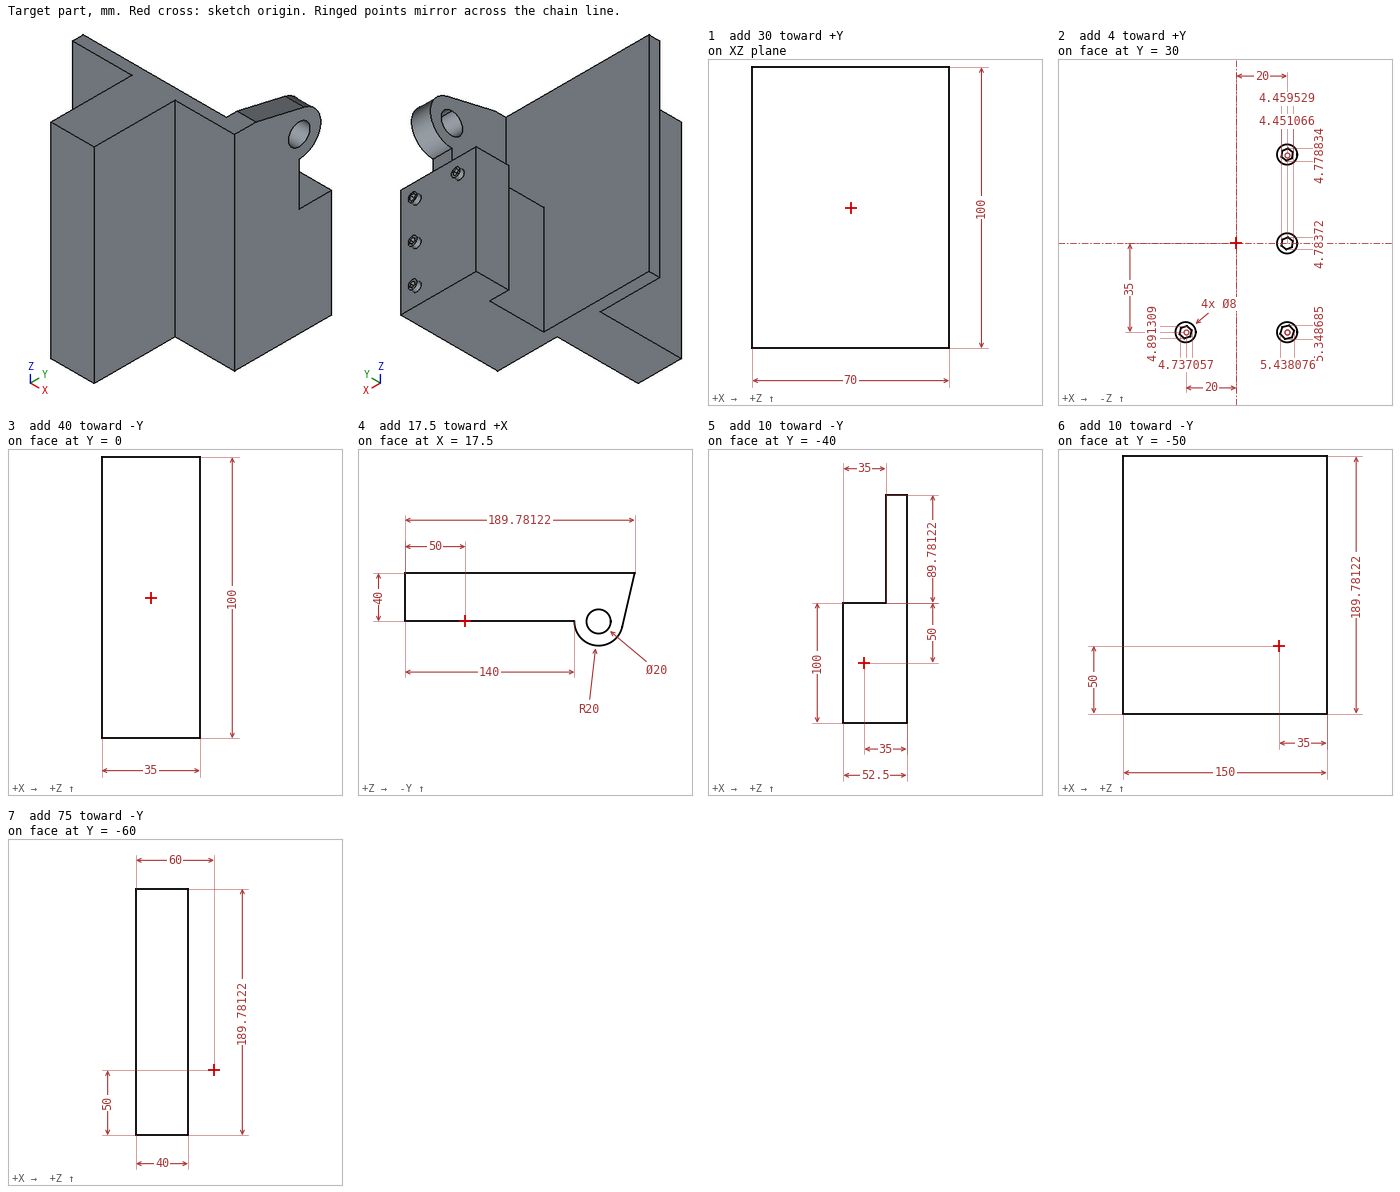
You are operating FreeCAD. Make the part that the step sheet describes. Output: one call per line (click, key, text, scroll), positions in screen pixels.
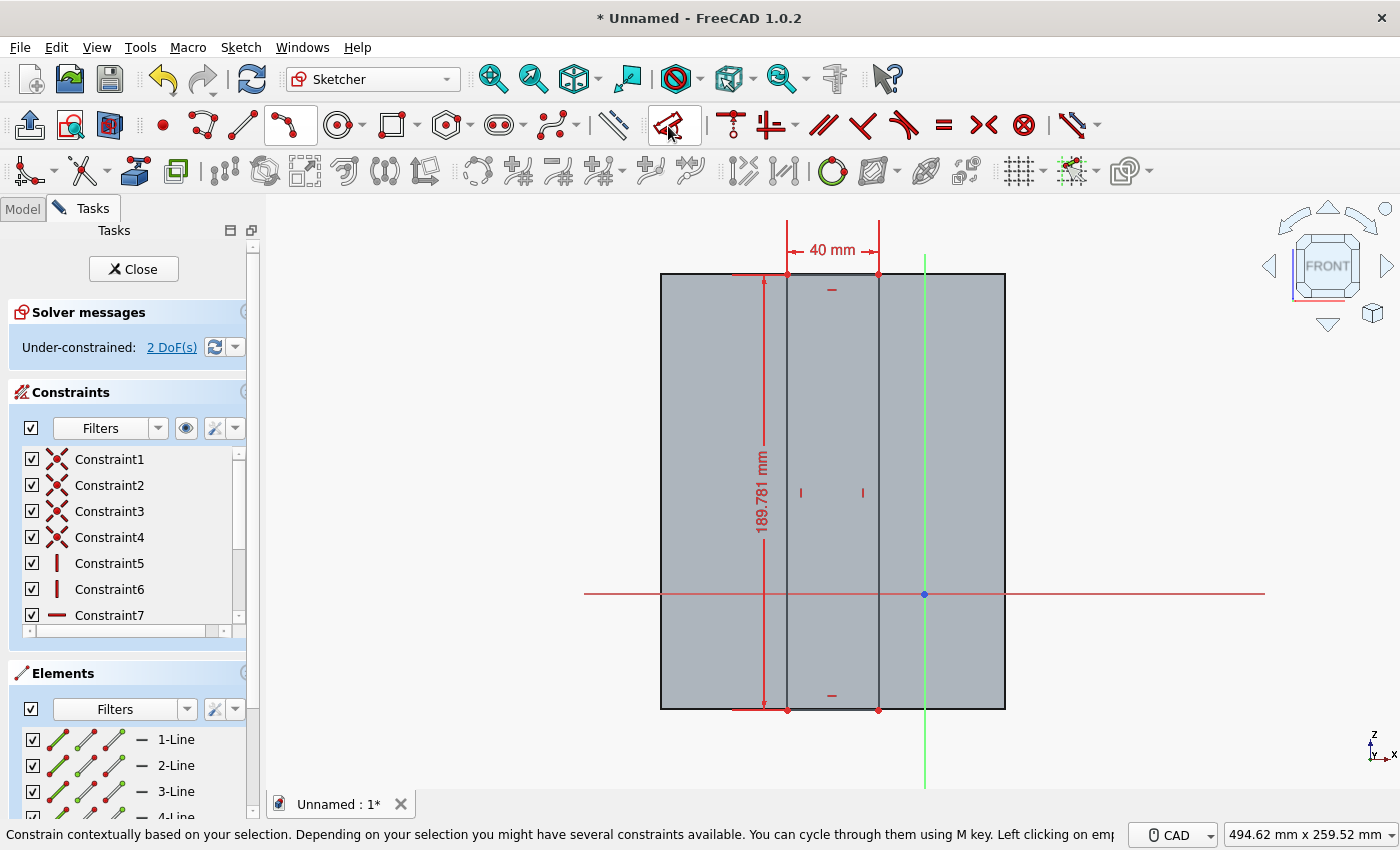
click(787, 275)
click(856, 241)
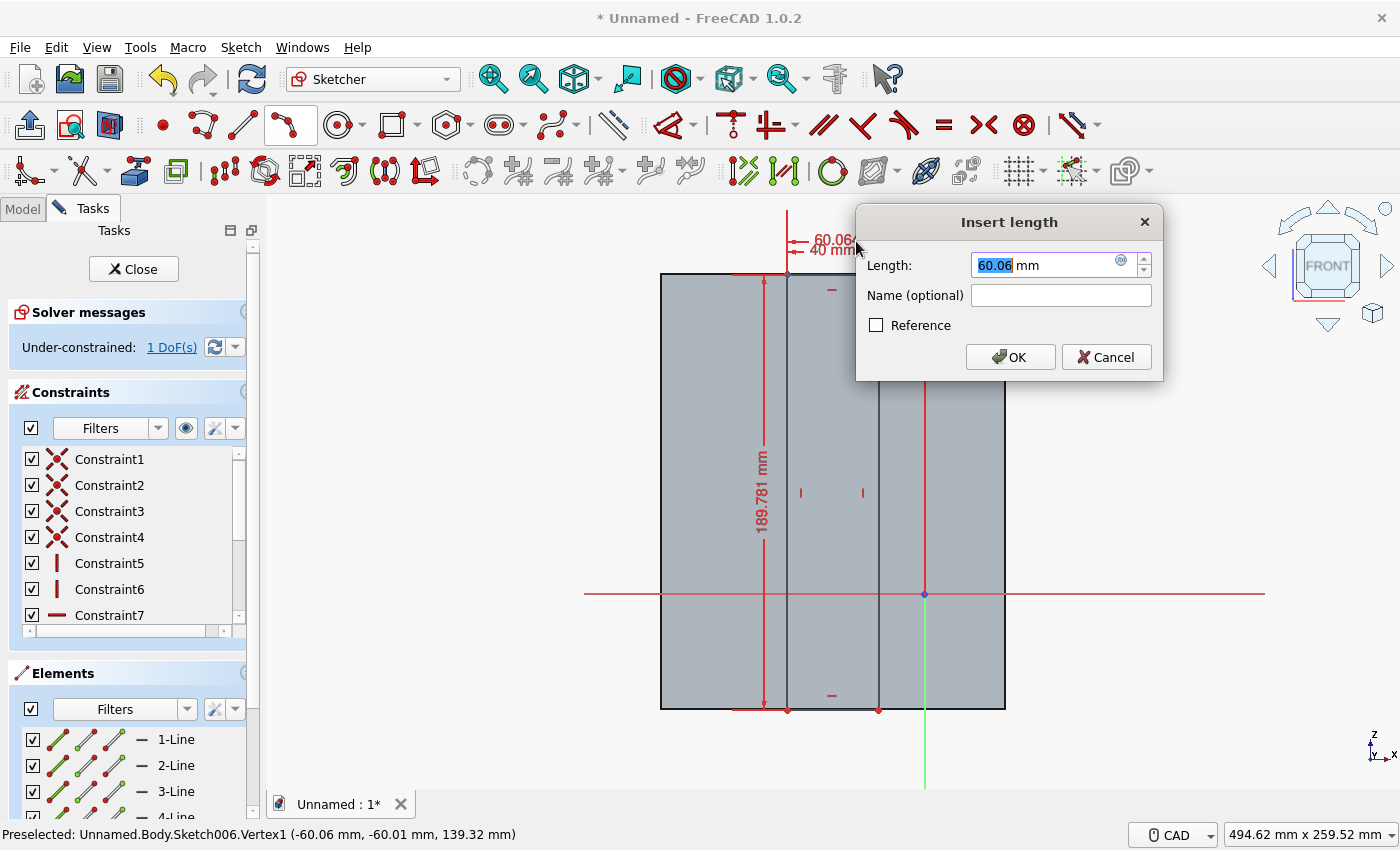
text(60)
key(Return)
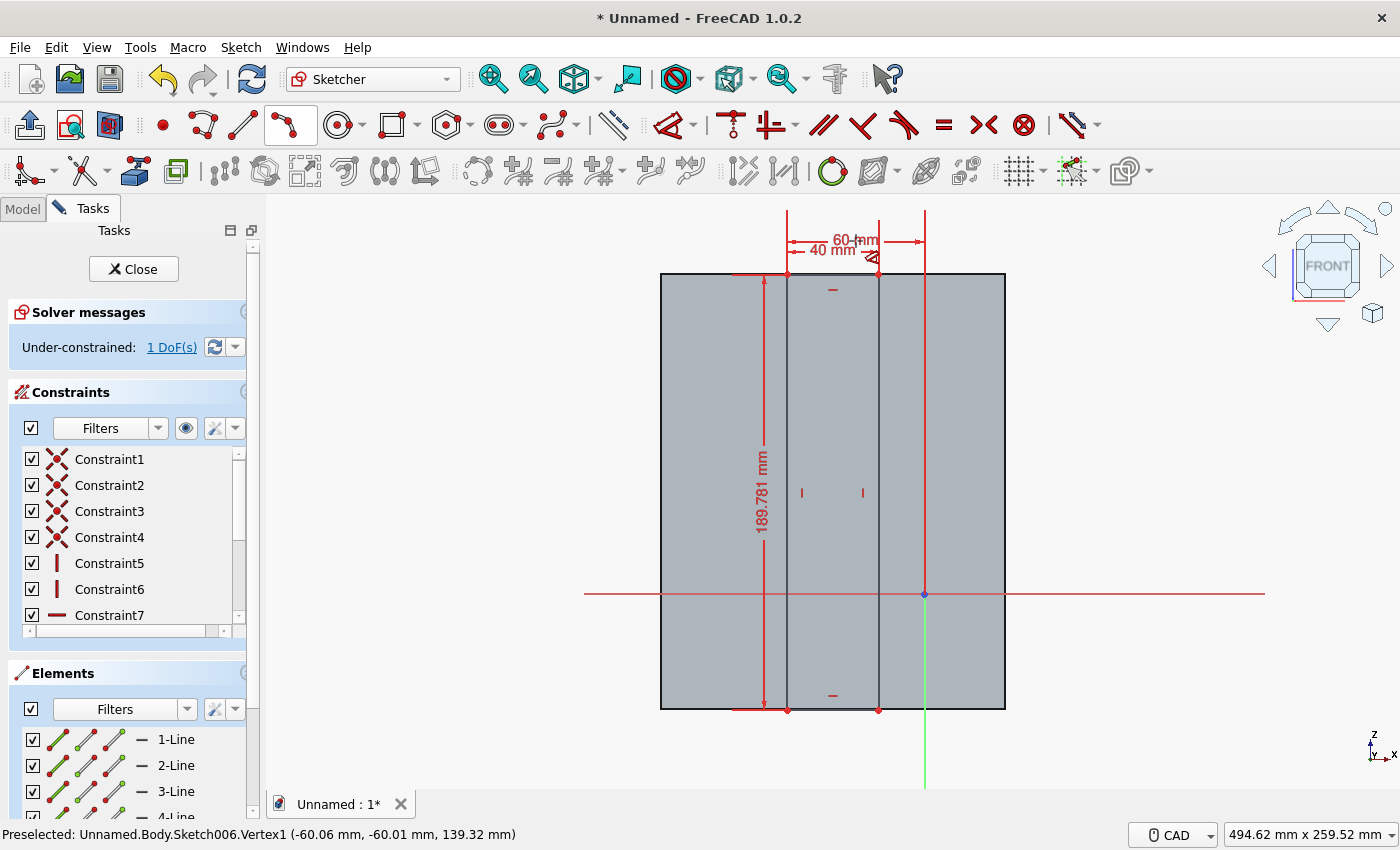
click(787, 710)
click(959, 652)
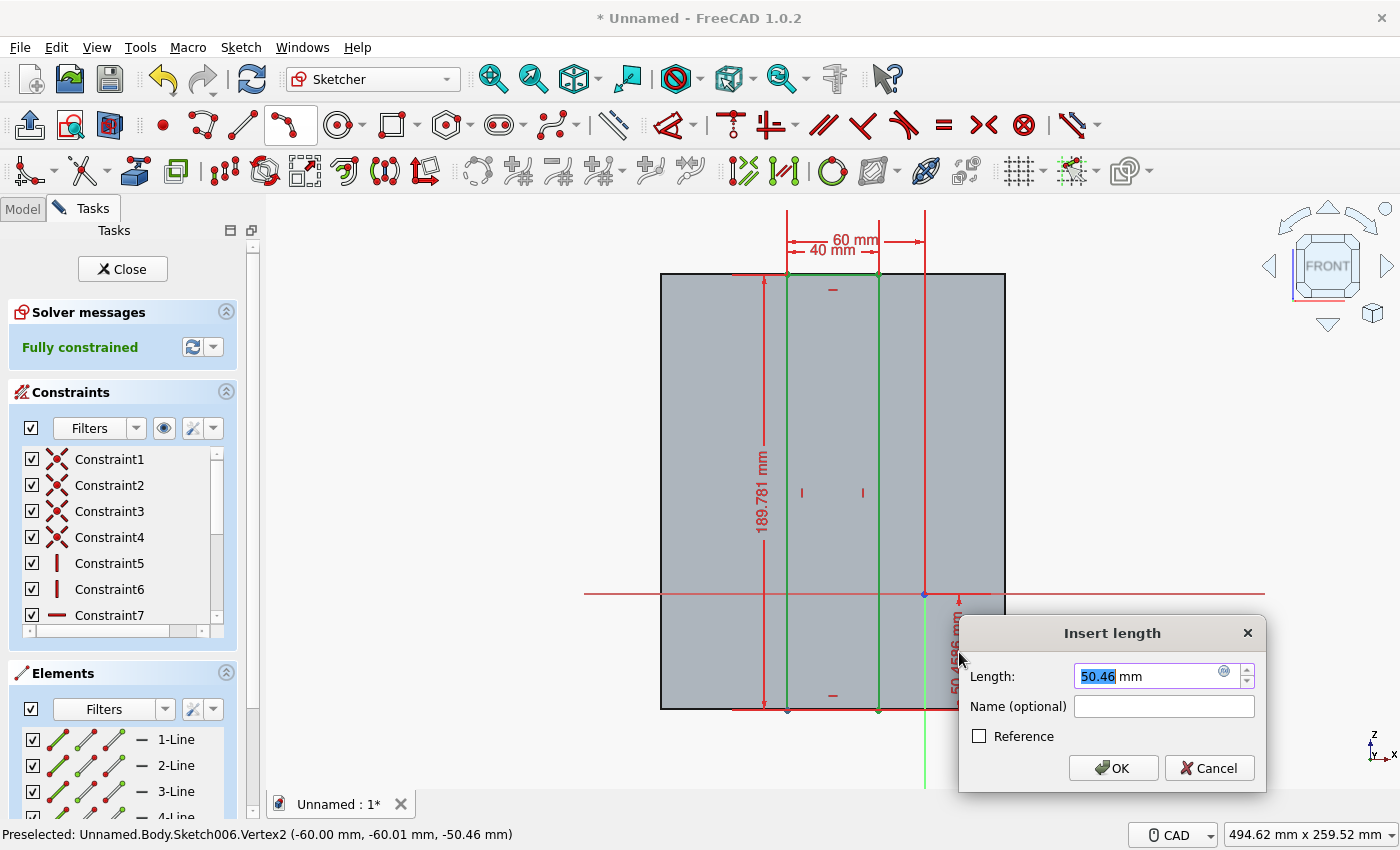
text(50)
key(Return)
key(Escape)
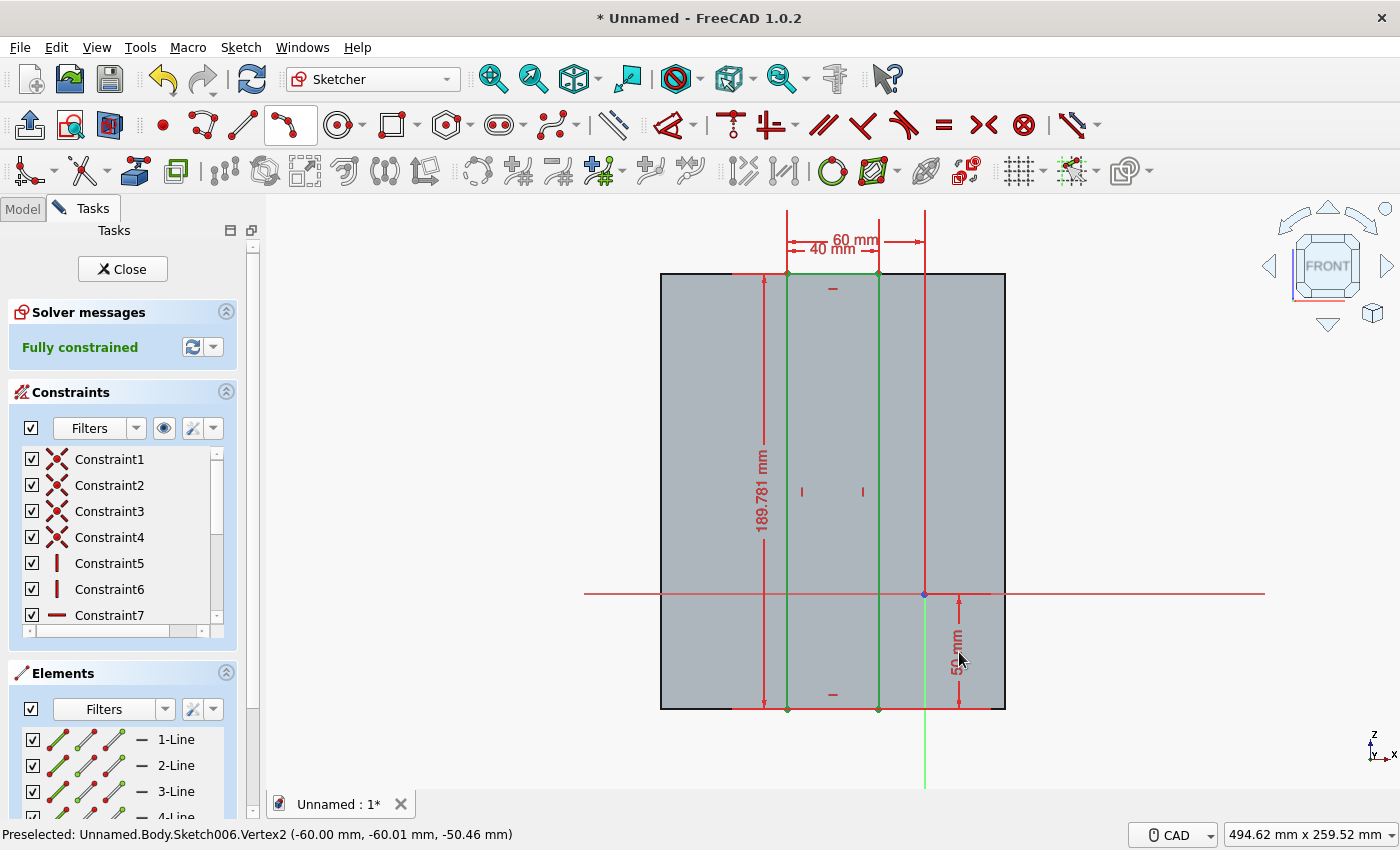
click(123, 269)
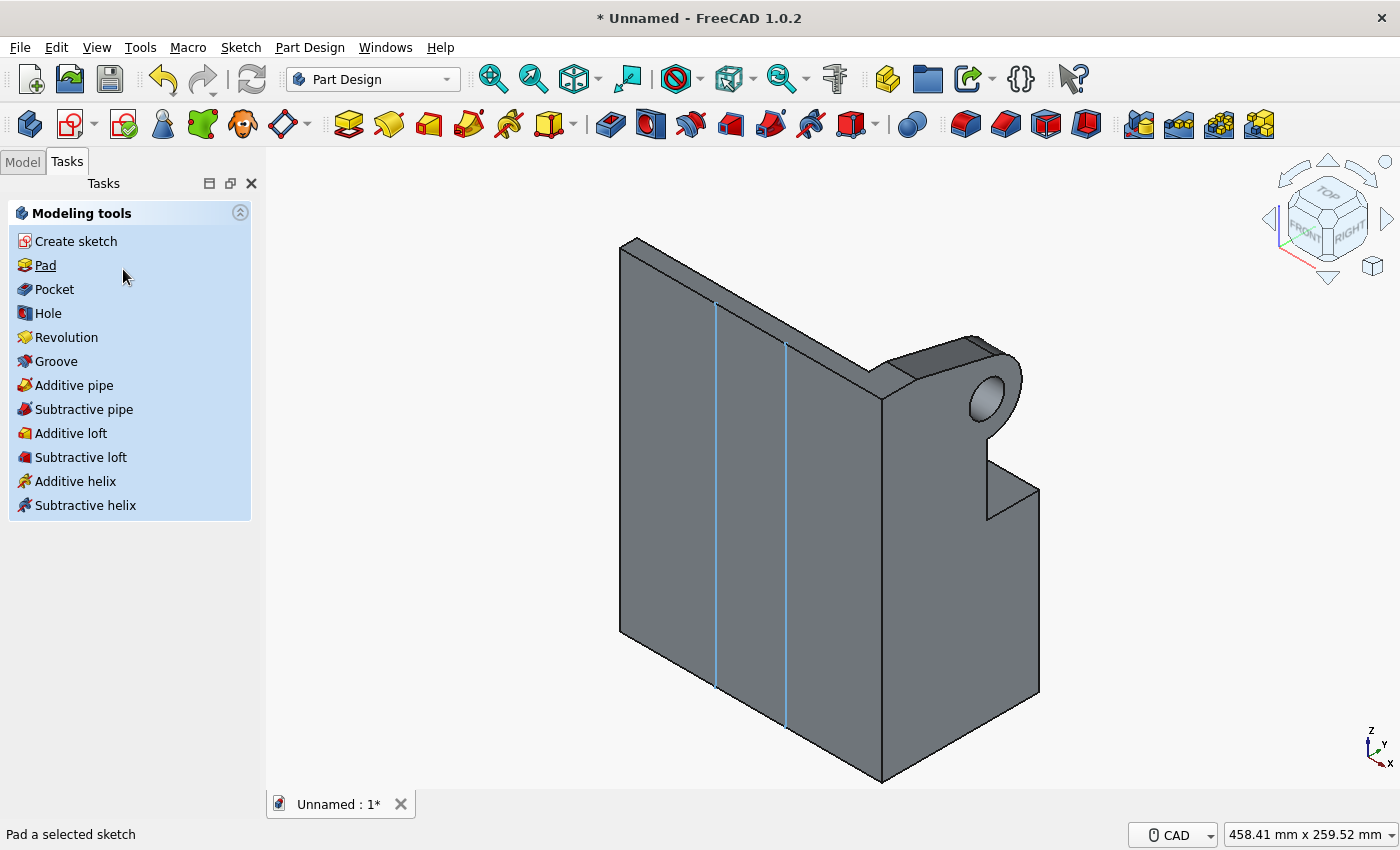
click(350, 124)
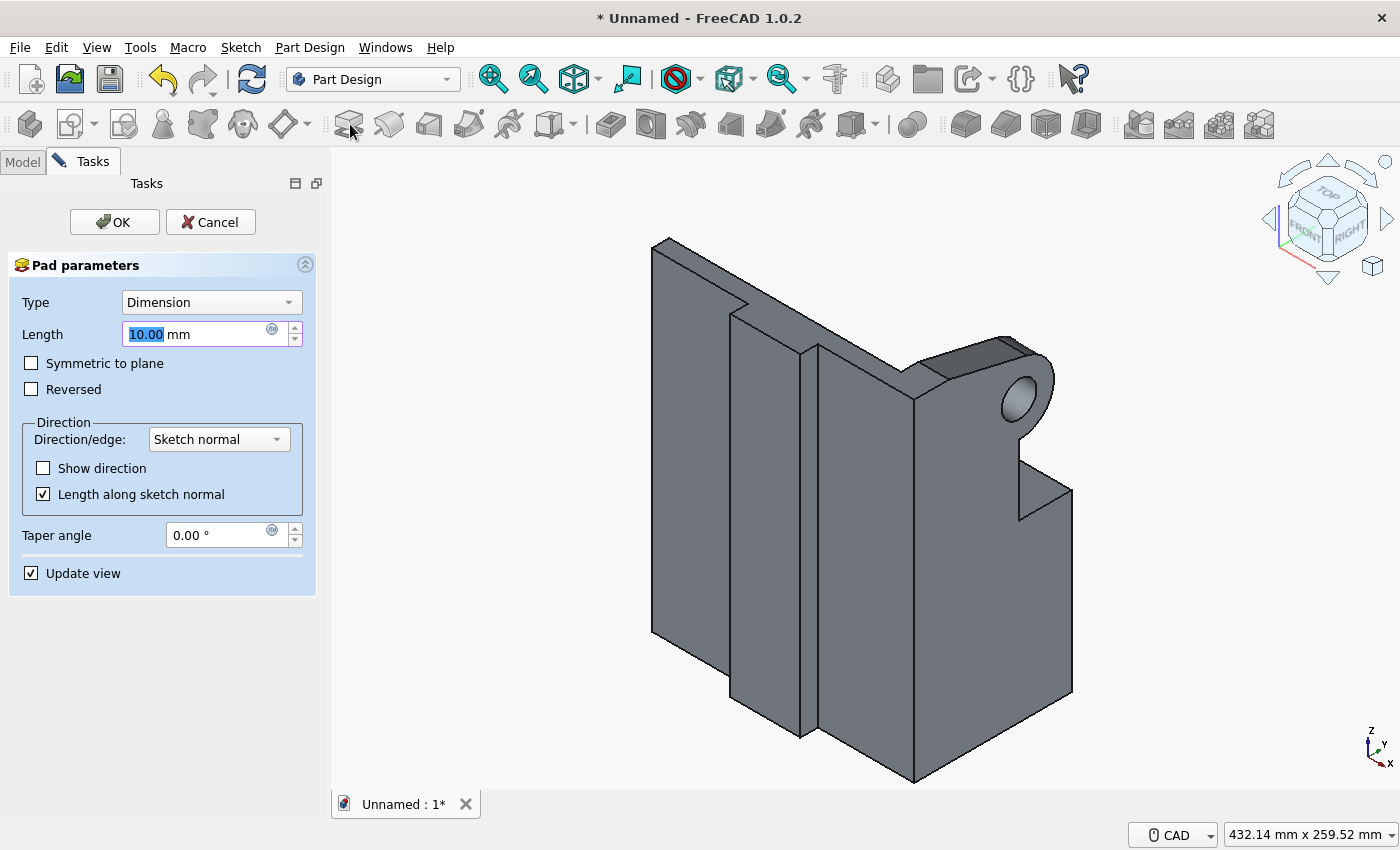
text(75)
key(Tab)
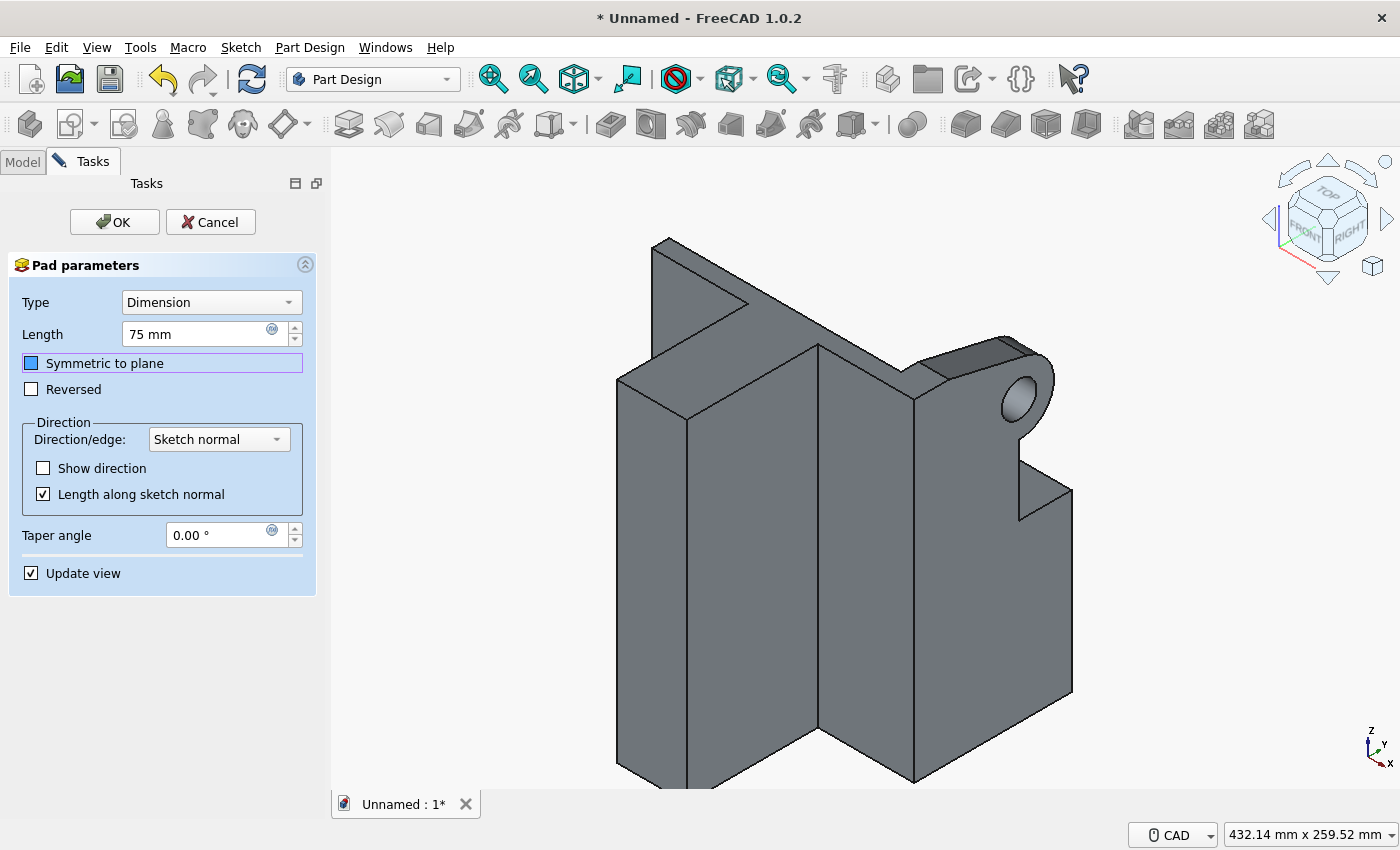
click(115, 222)